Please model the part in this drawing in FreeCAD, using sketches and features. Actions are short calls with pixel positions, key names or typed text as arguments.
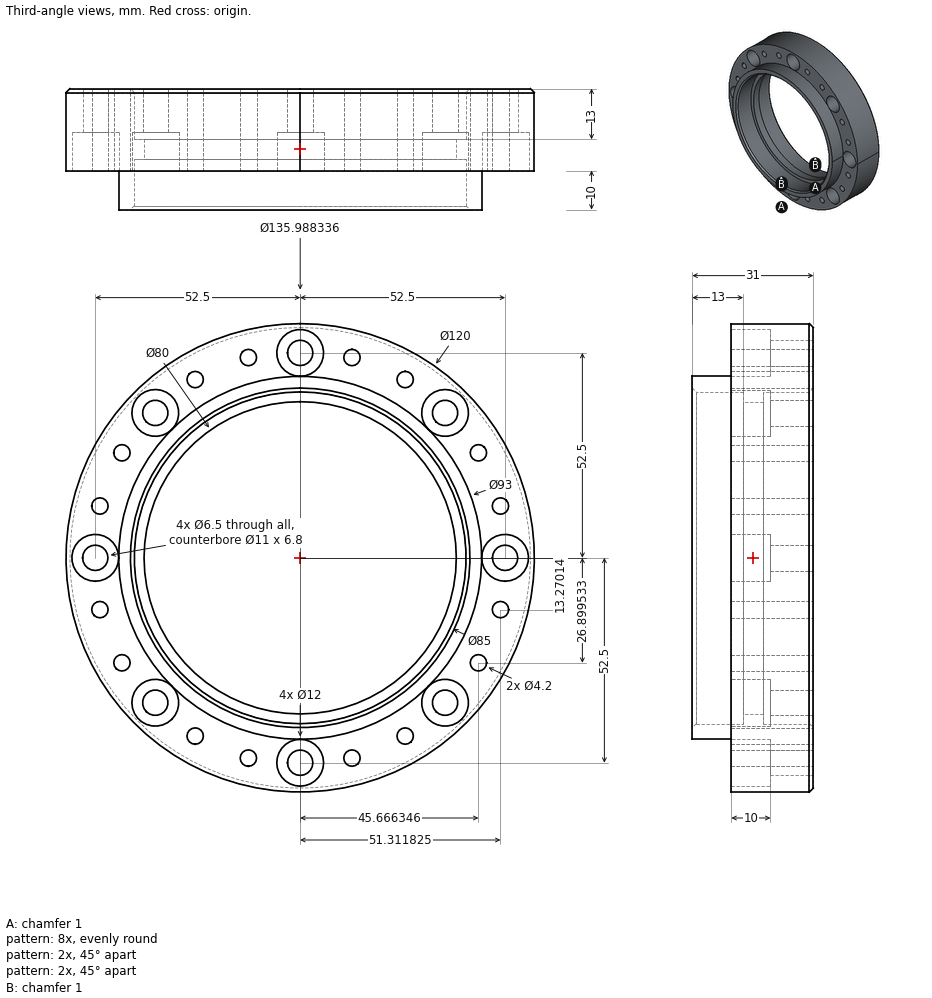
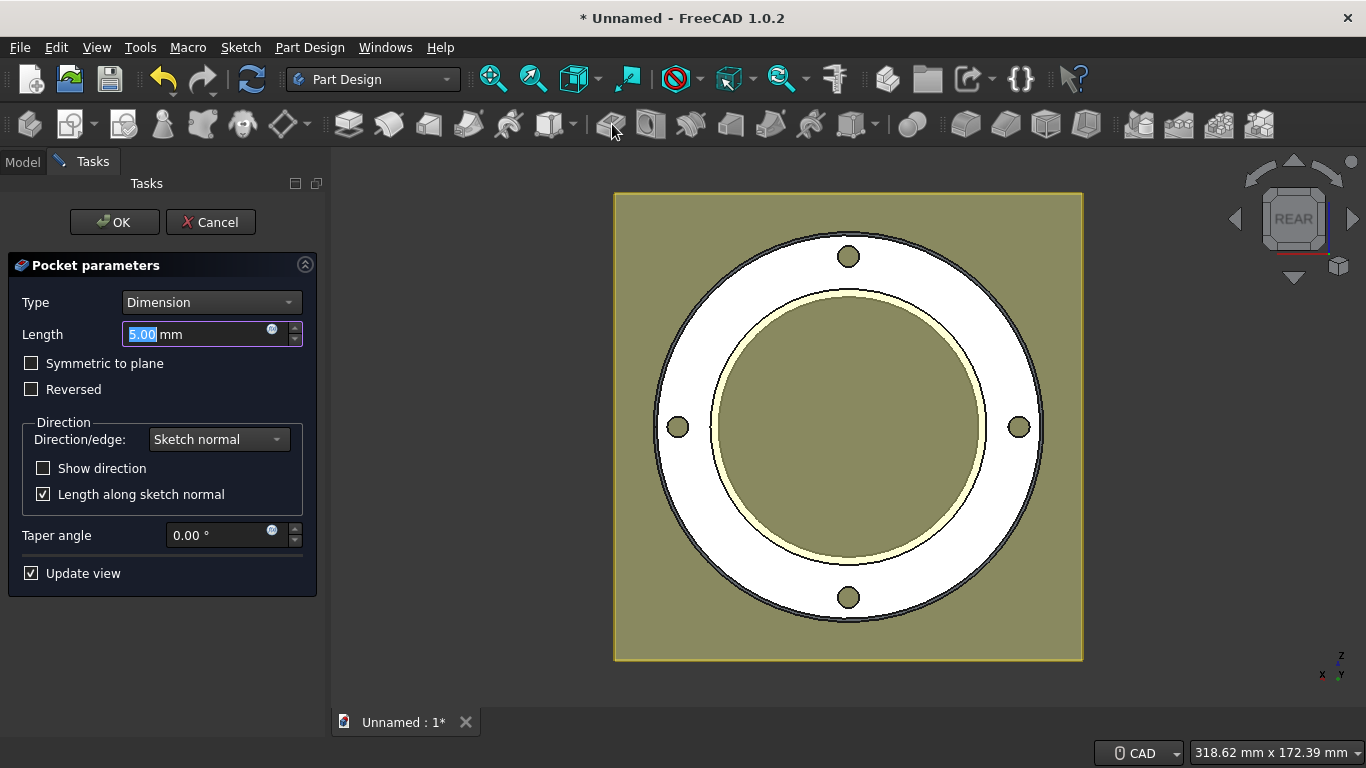
text(13)
key(Tab)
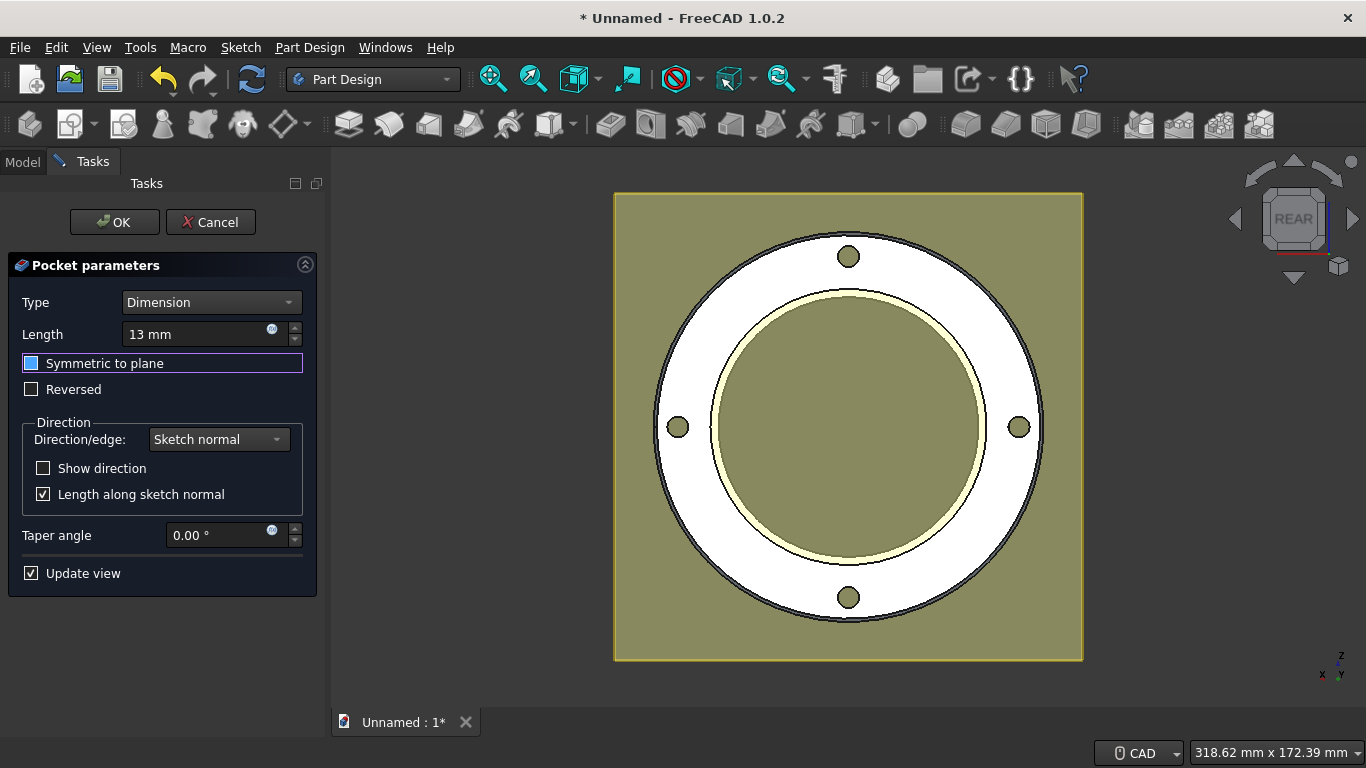
click(30, 389)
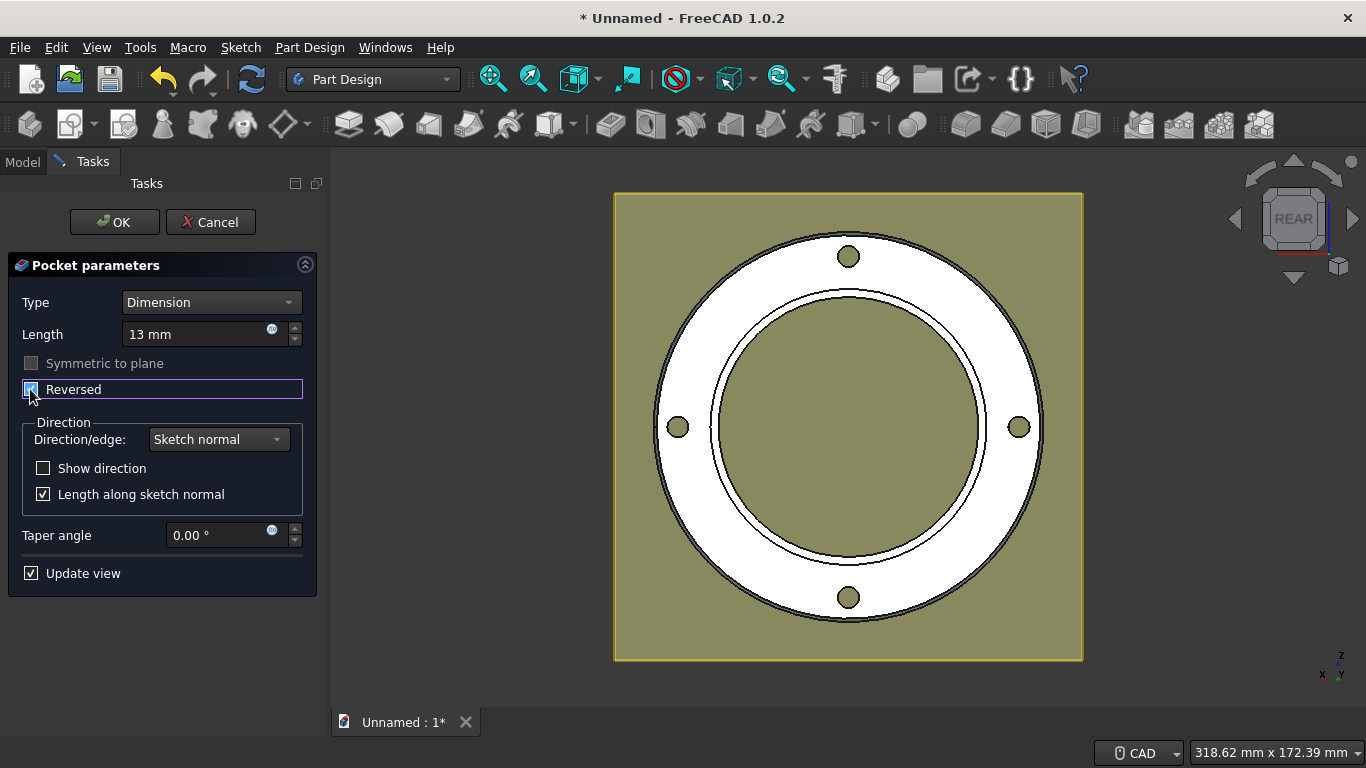
click(115, 222)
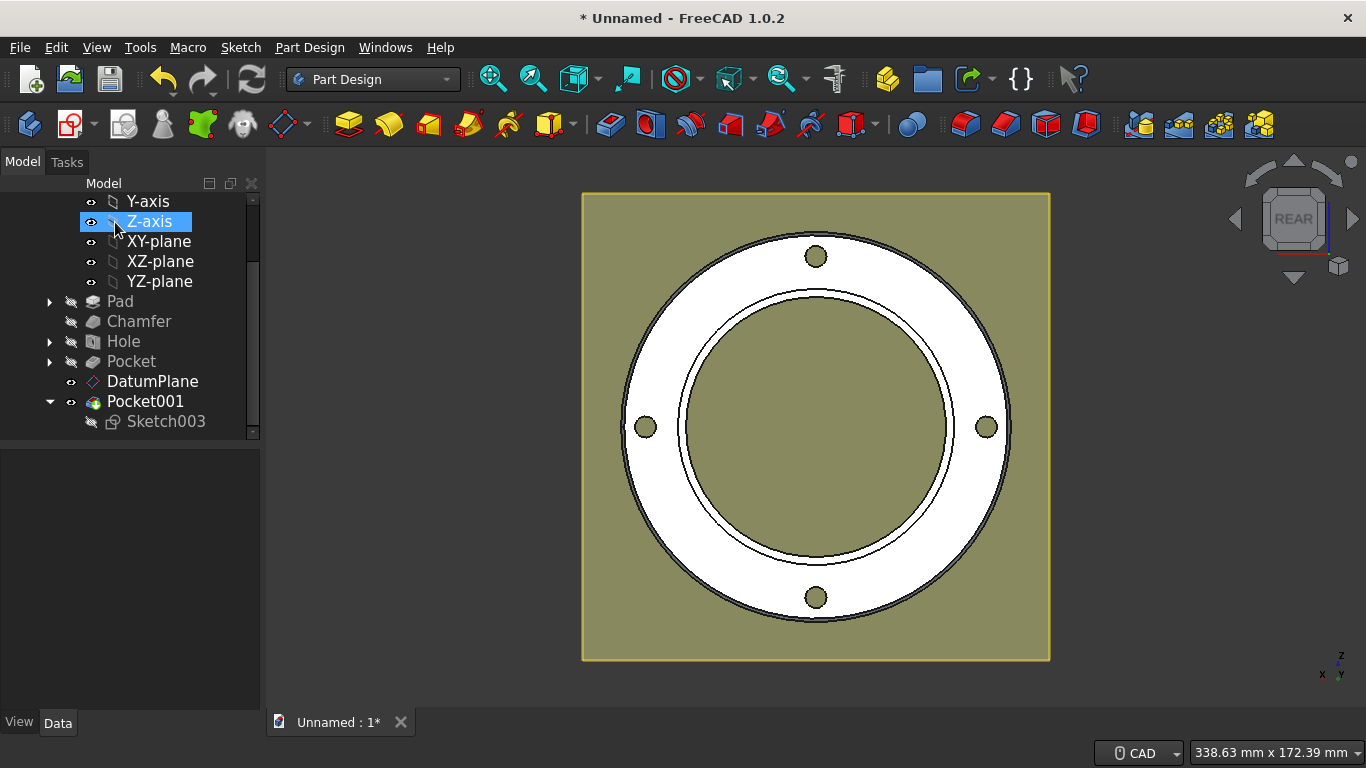
click(116, 382)
key(space)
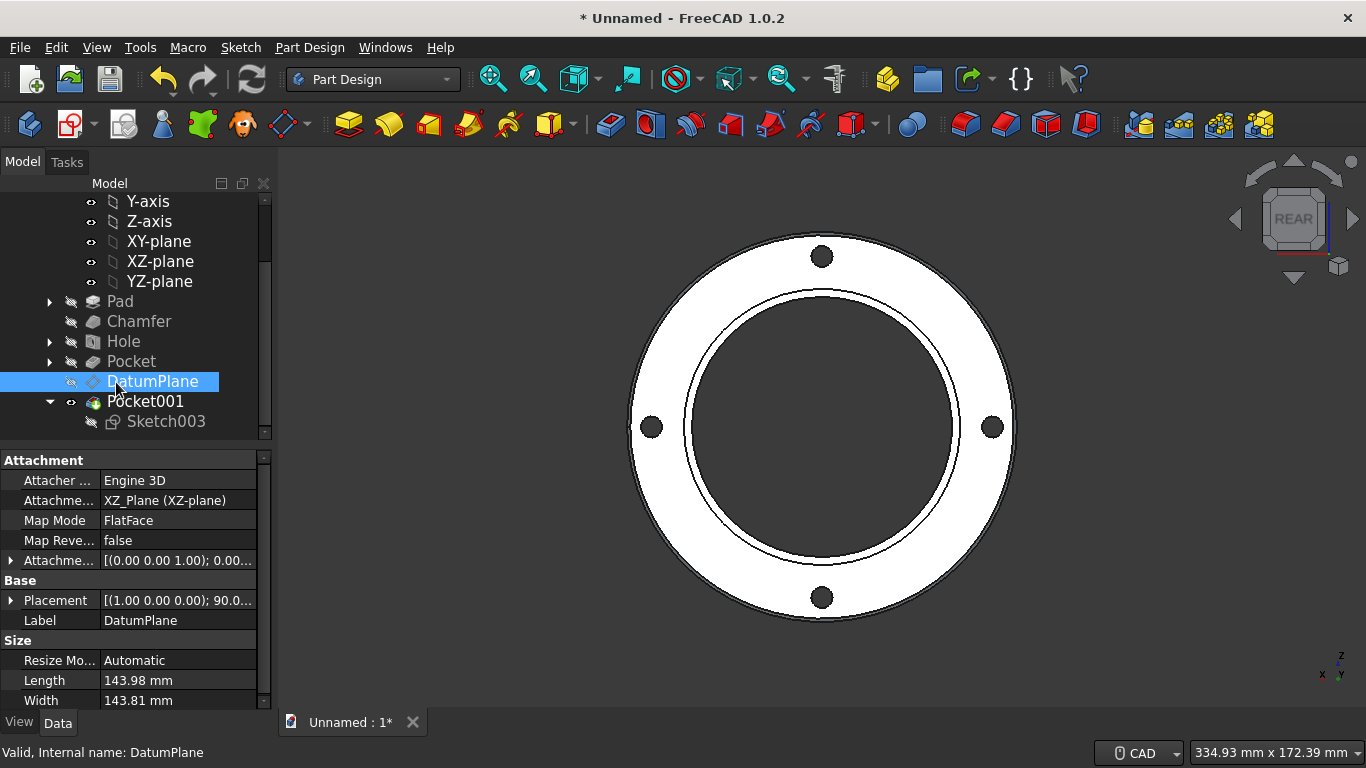
key(0)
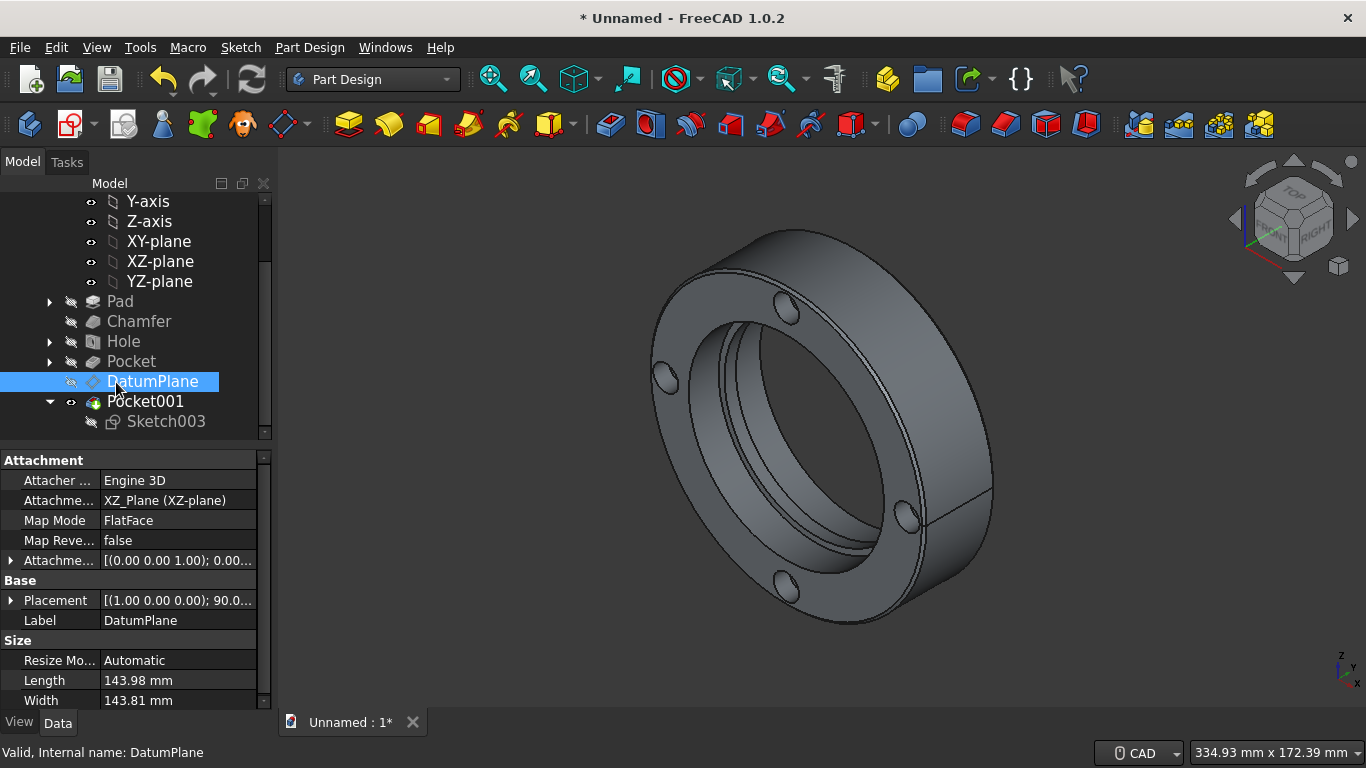
click(748, 290)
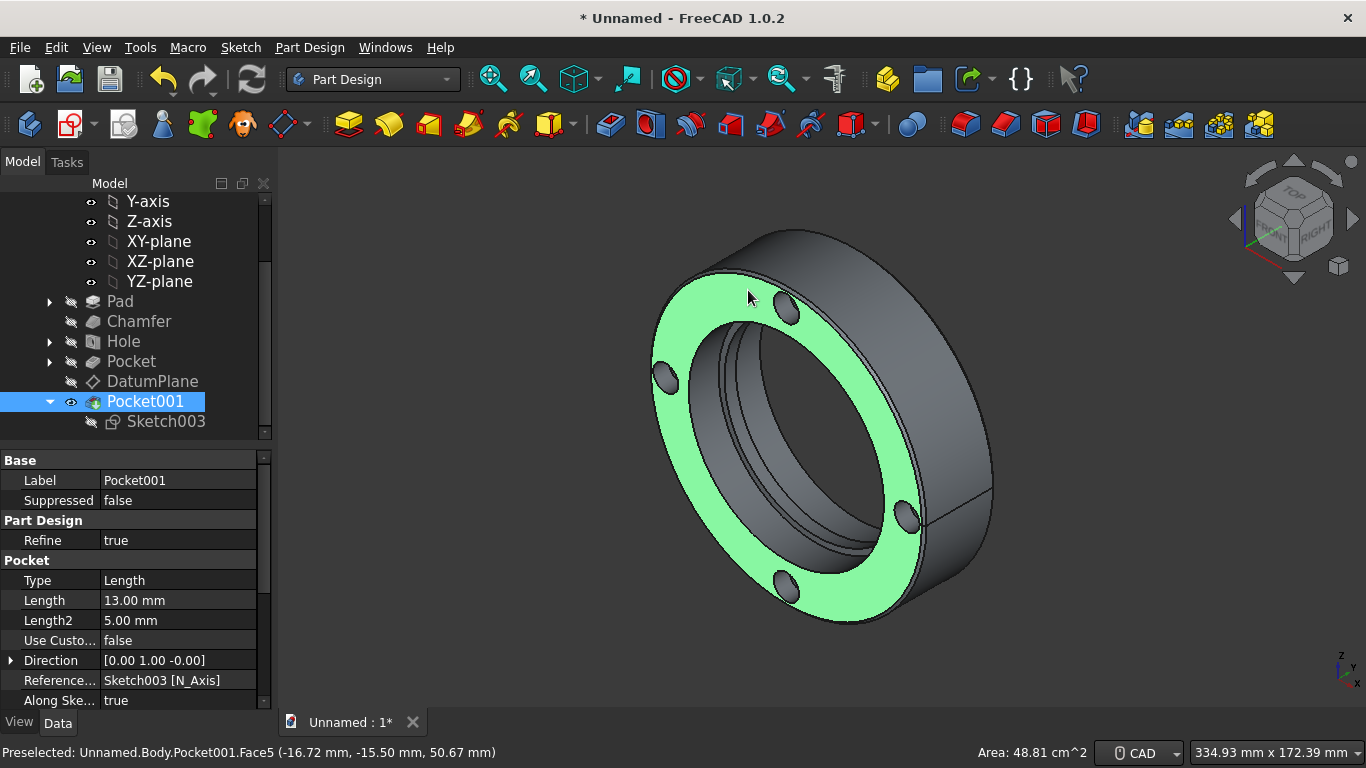
click(70, 124)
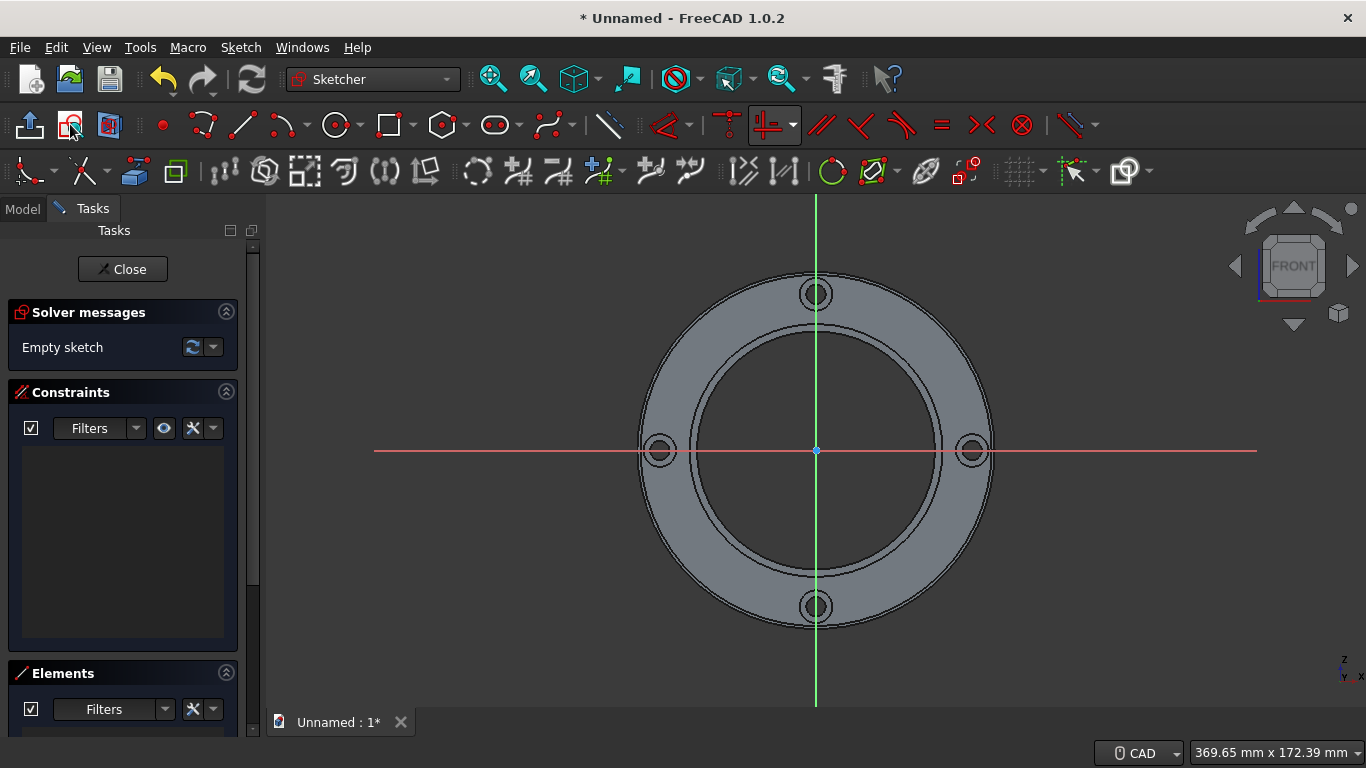
click(336, 126)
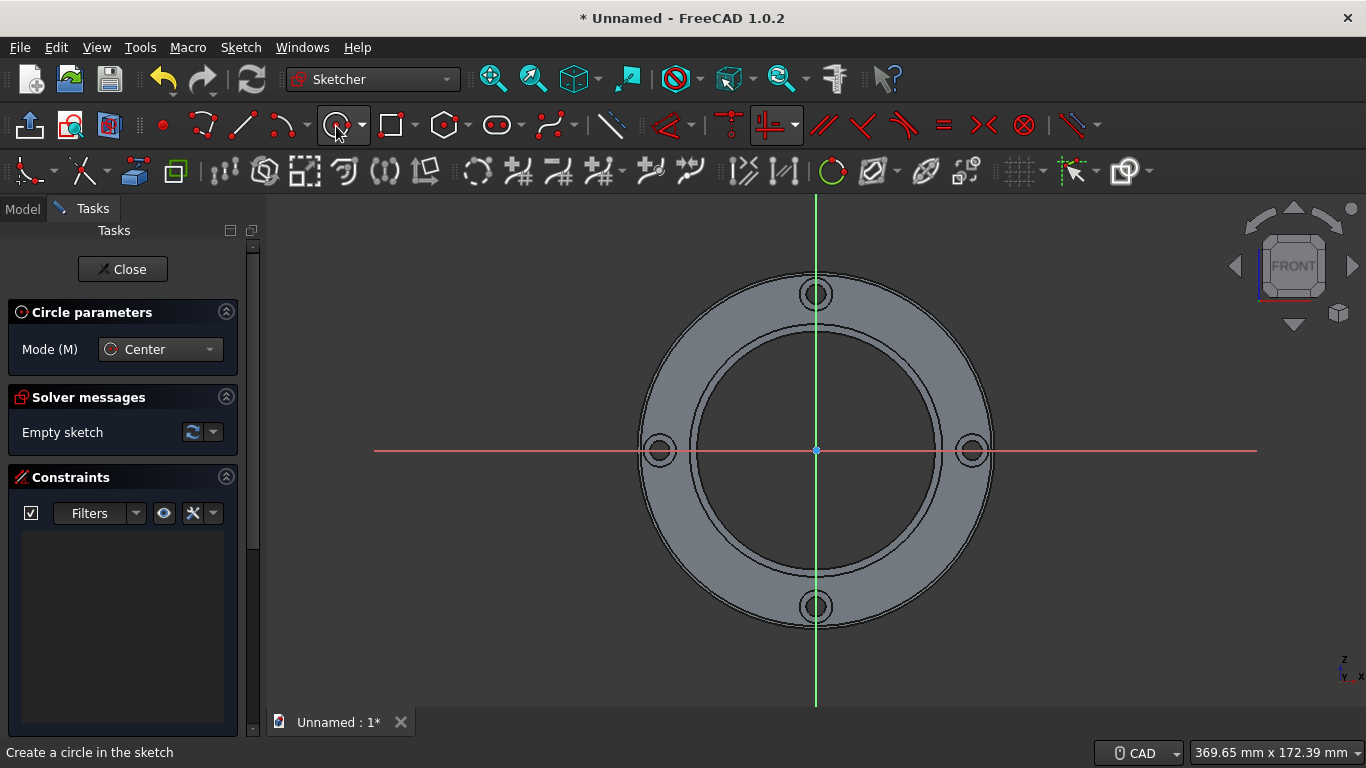
click(816, 451)
move(959, 307)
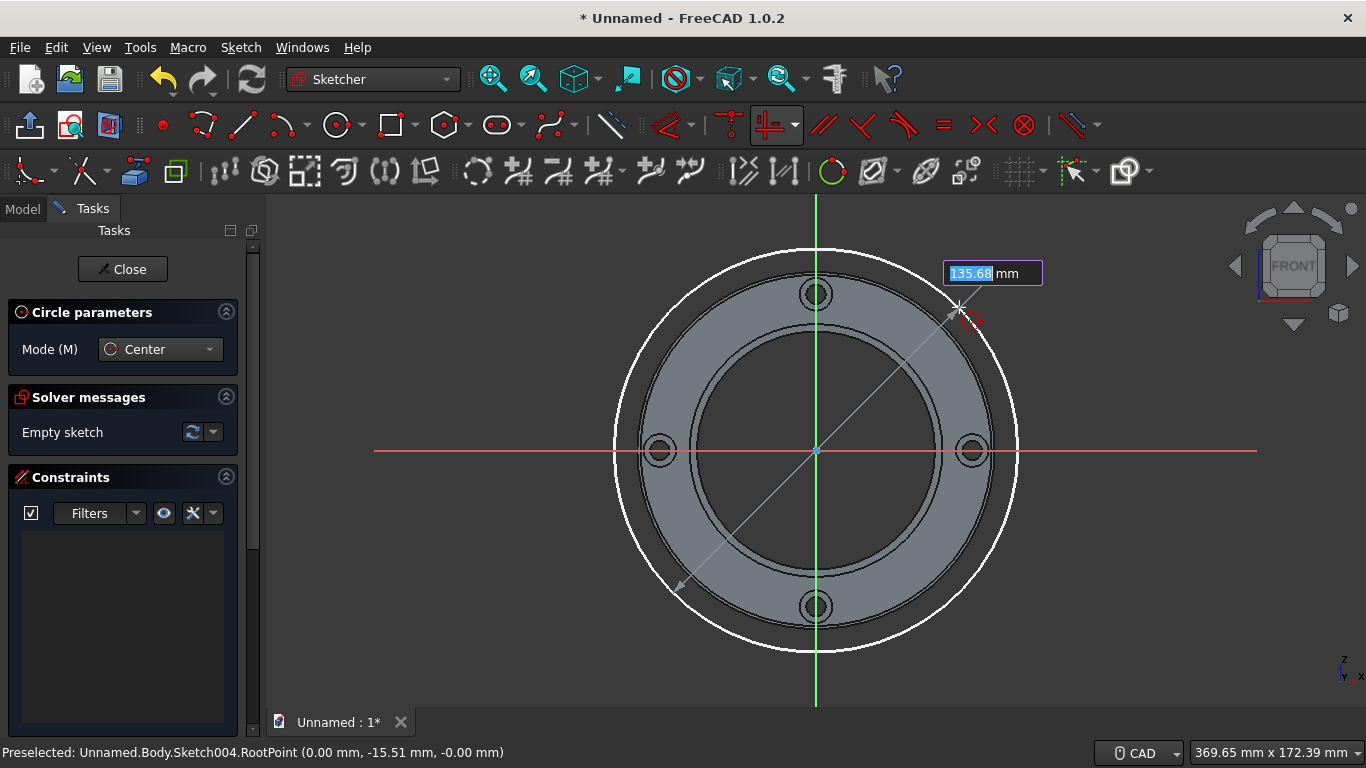
text(135.988336)
key(Return)